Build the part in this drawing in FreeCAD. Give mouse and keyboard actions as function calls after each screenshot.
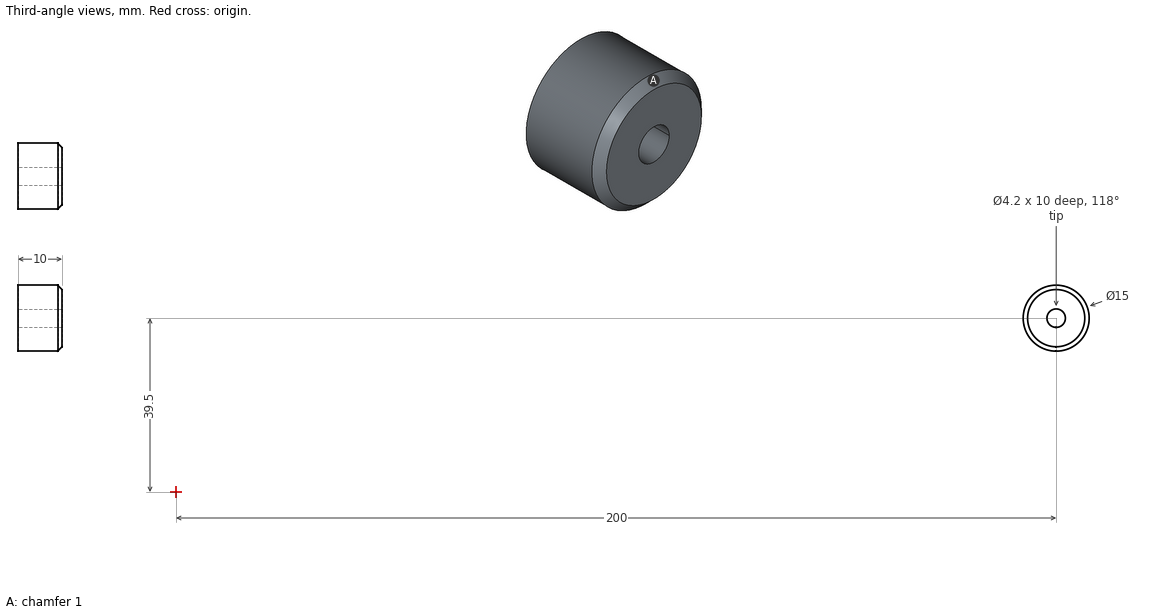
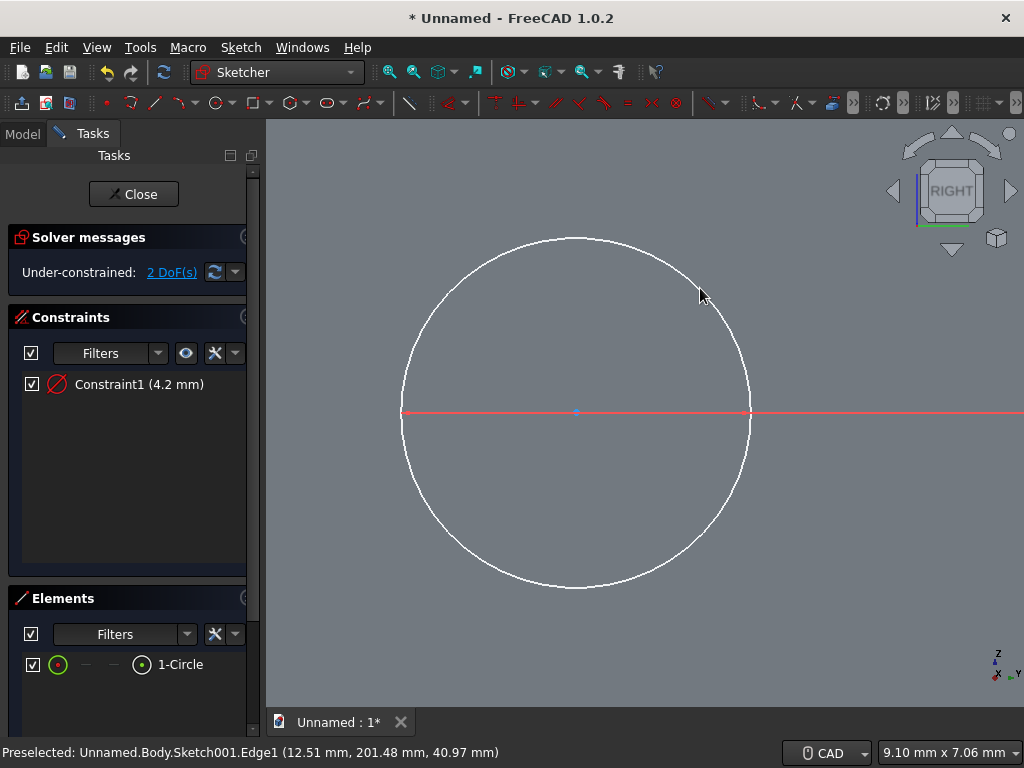
click(448, 104)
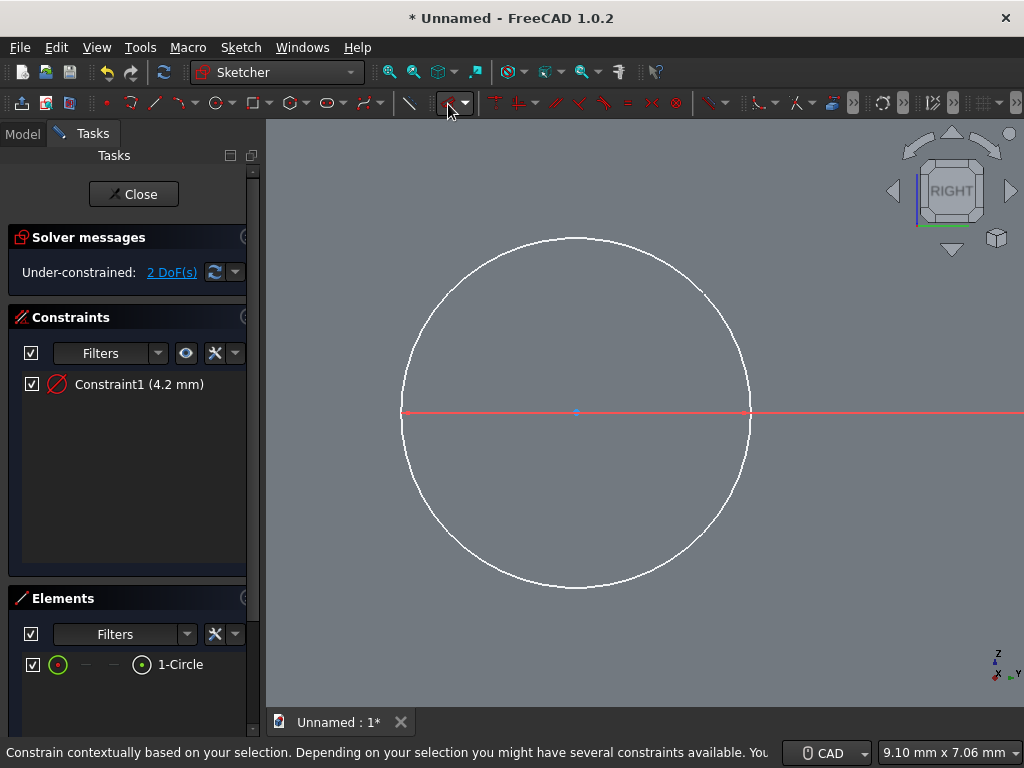
click(576, 413)
click(435, 379)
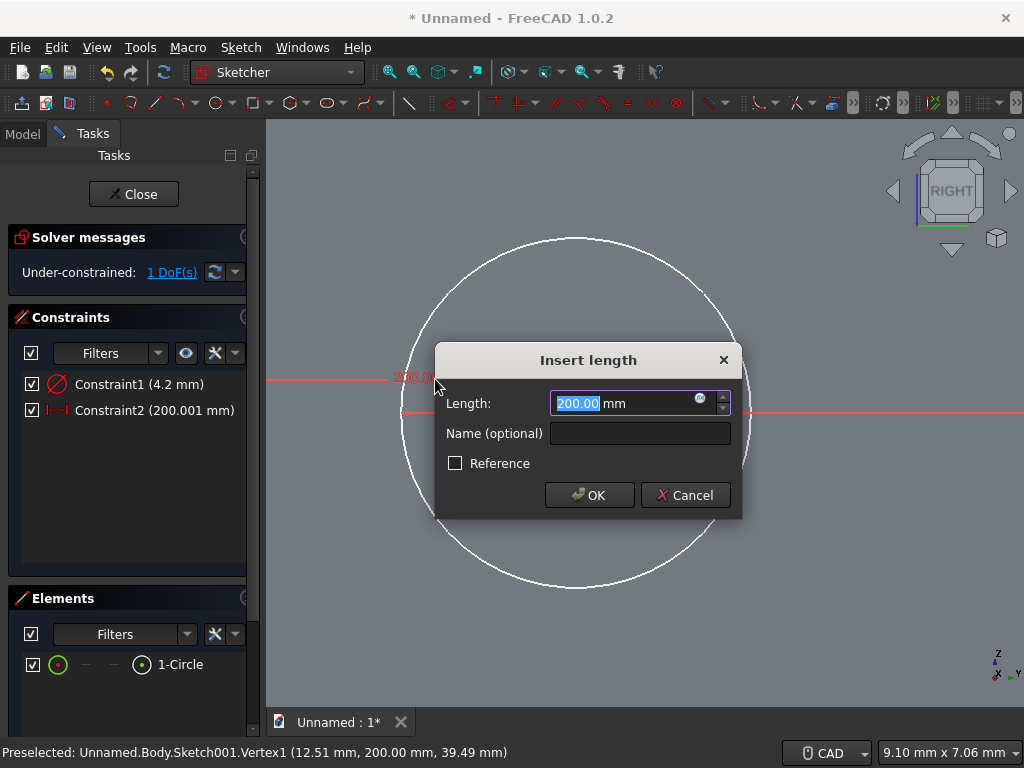
text(200)
key(Return)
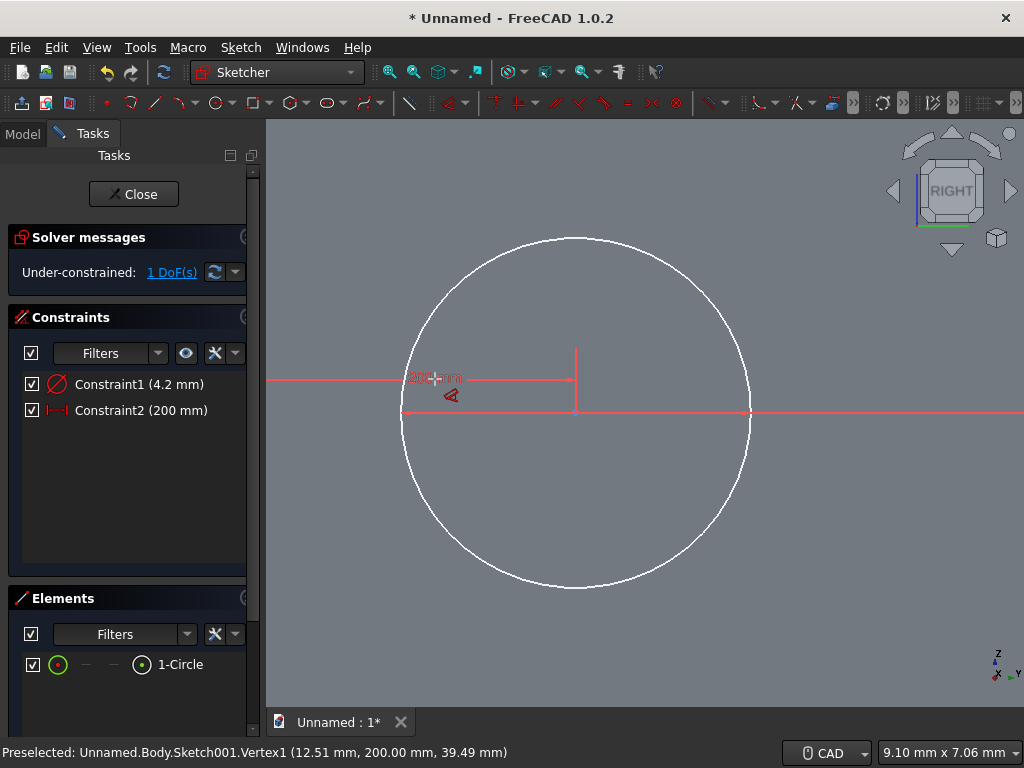
click(576, 413)
click(610, 546)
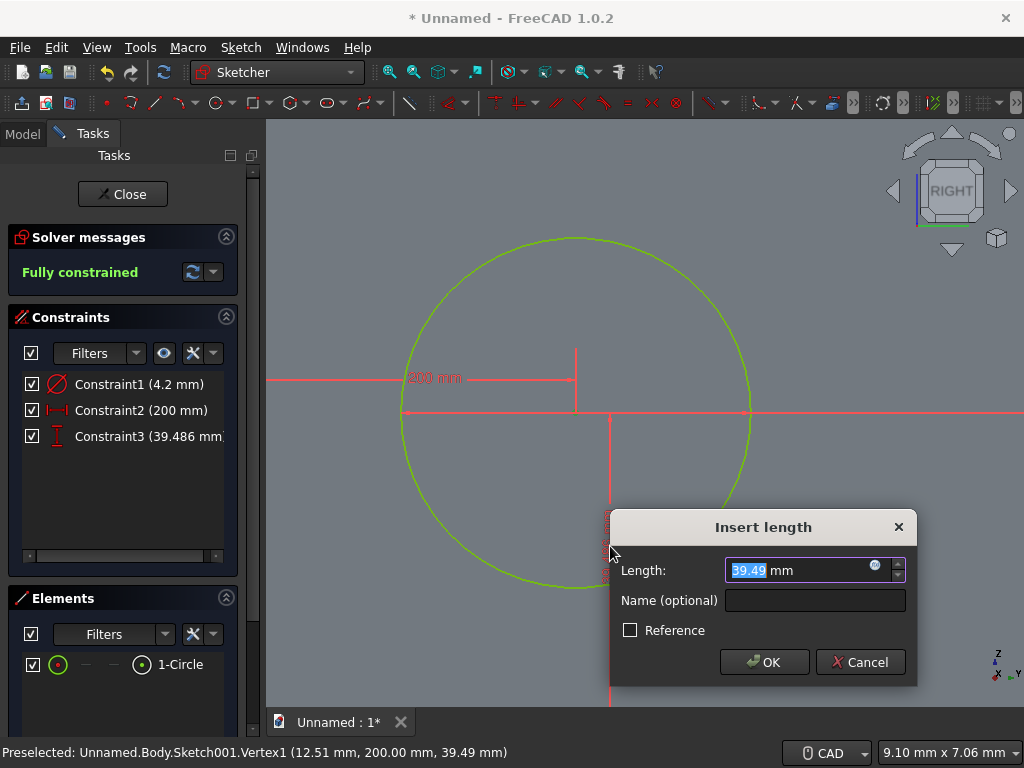
text(39.5)
key(Return)
key(Escape)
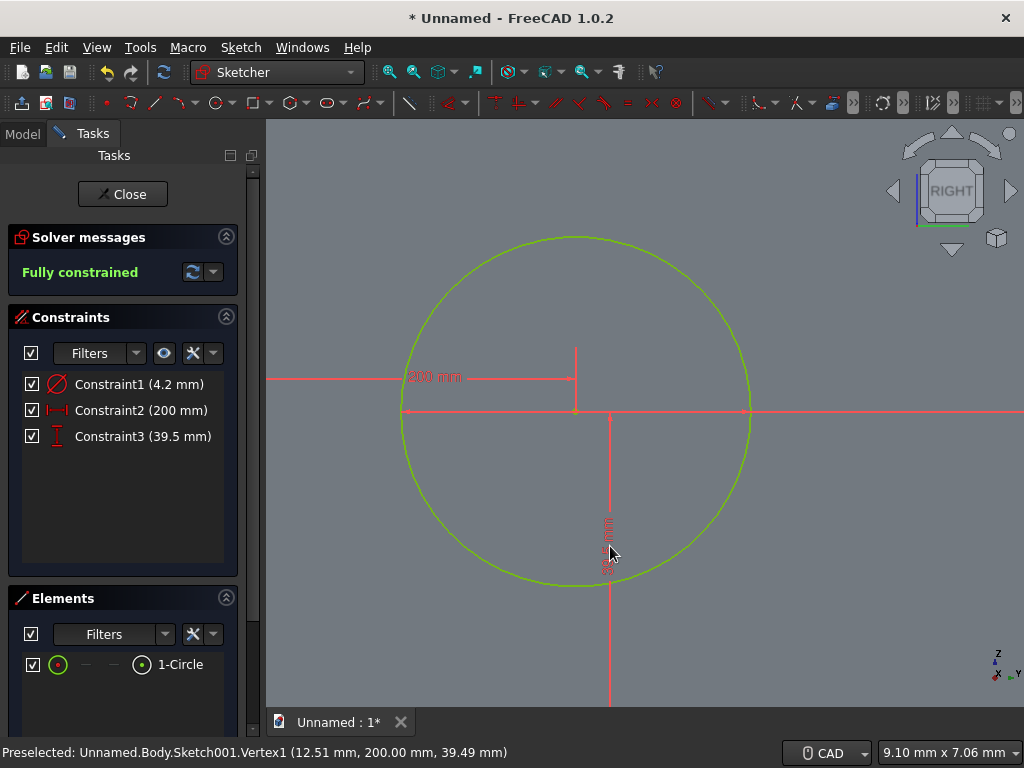
click(123, 194)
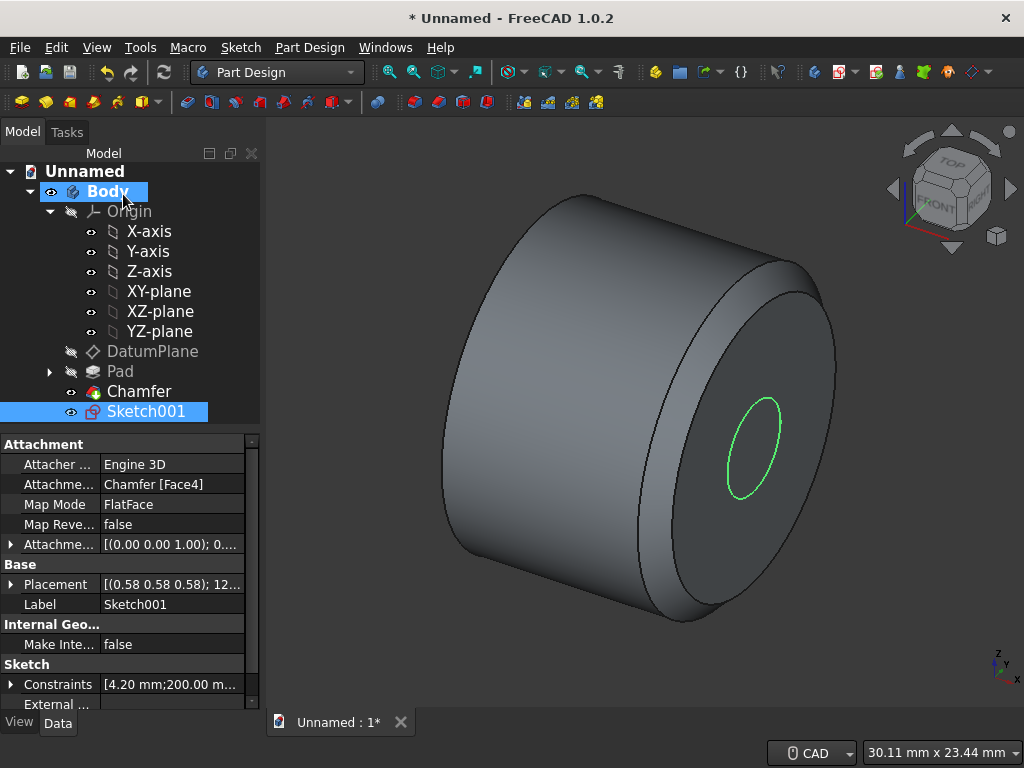
click(212, 102)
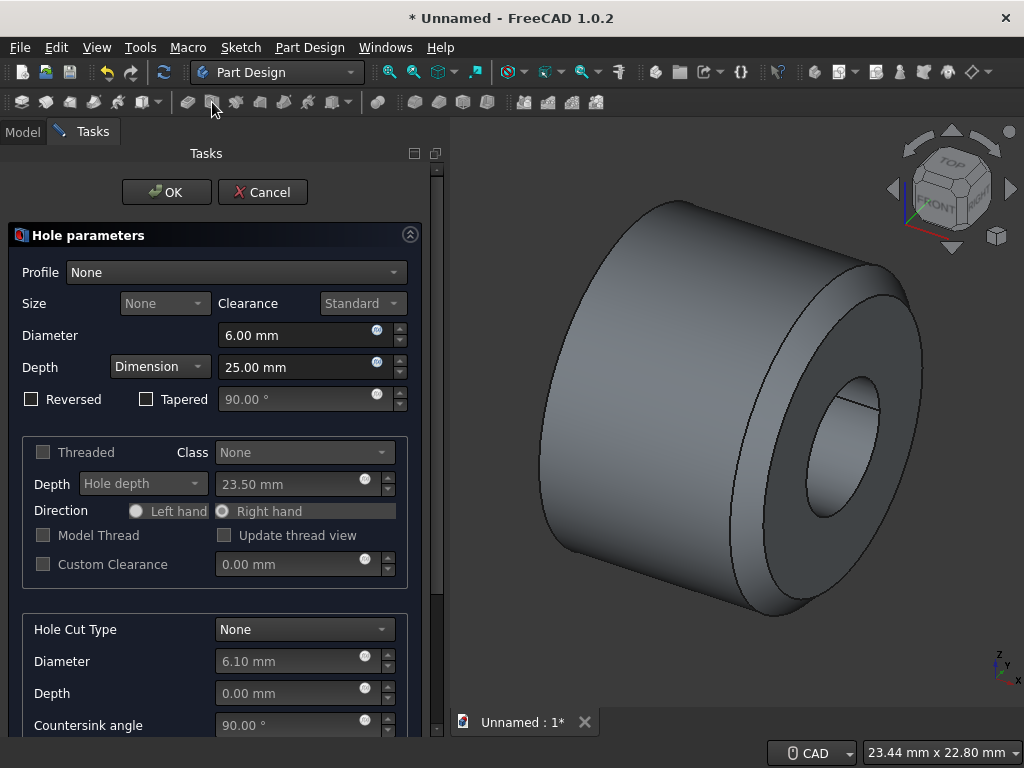
triple_click(305, 335)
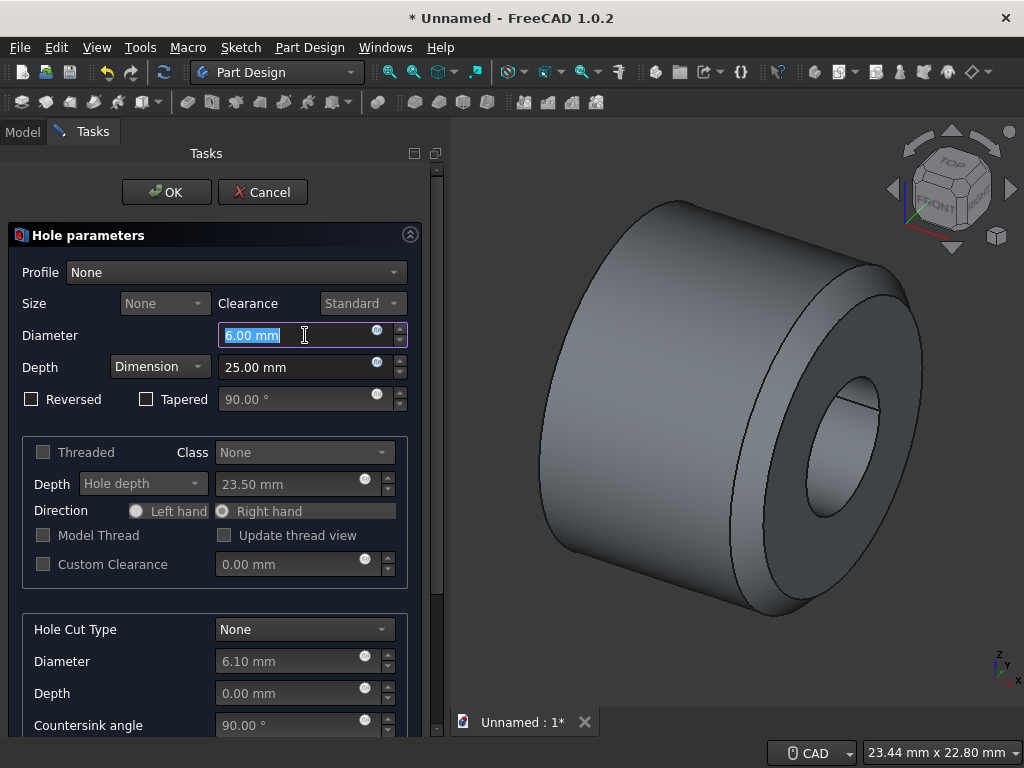
text(4.2)
key(Tab)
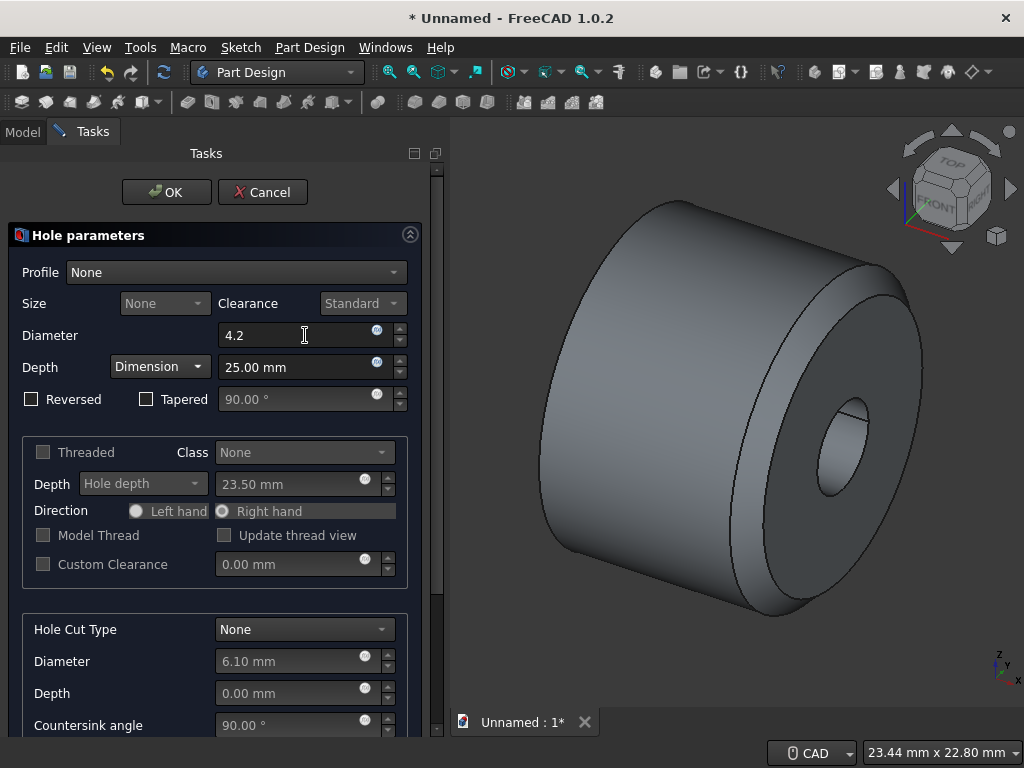
triple_click(305, 367)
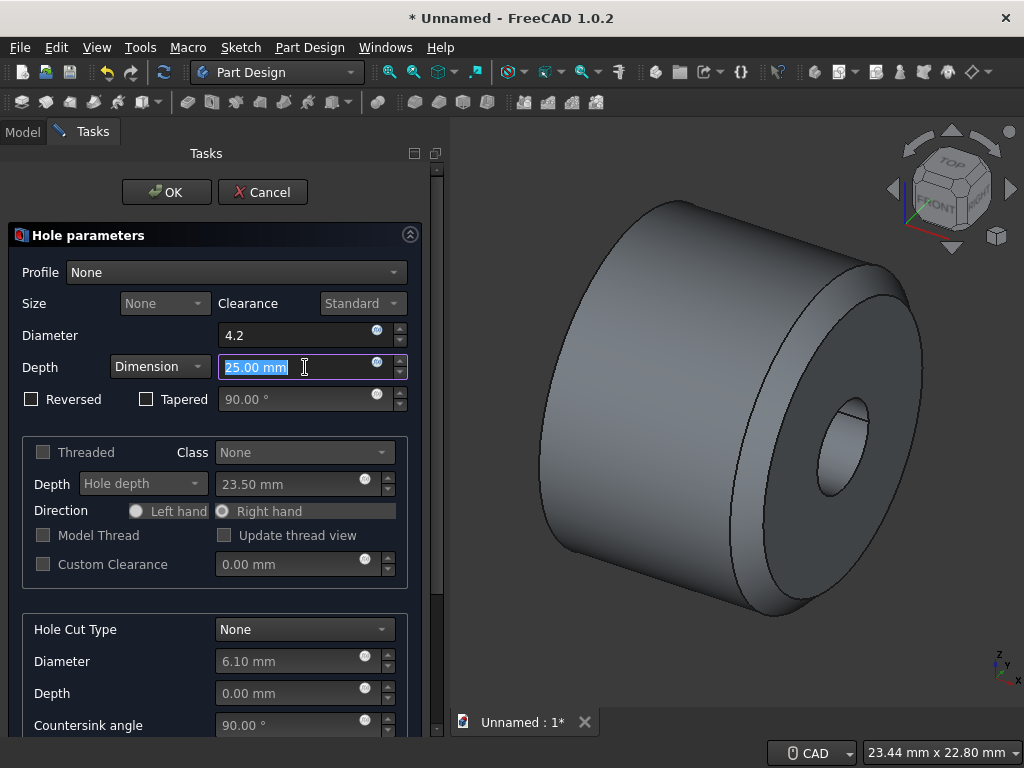
text(10)
key(Tab)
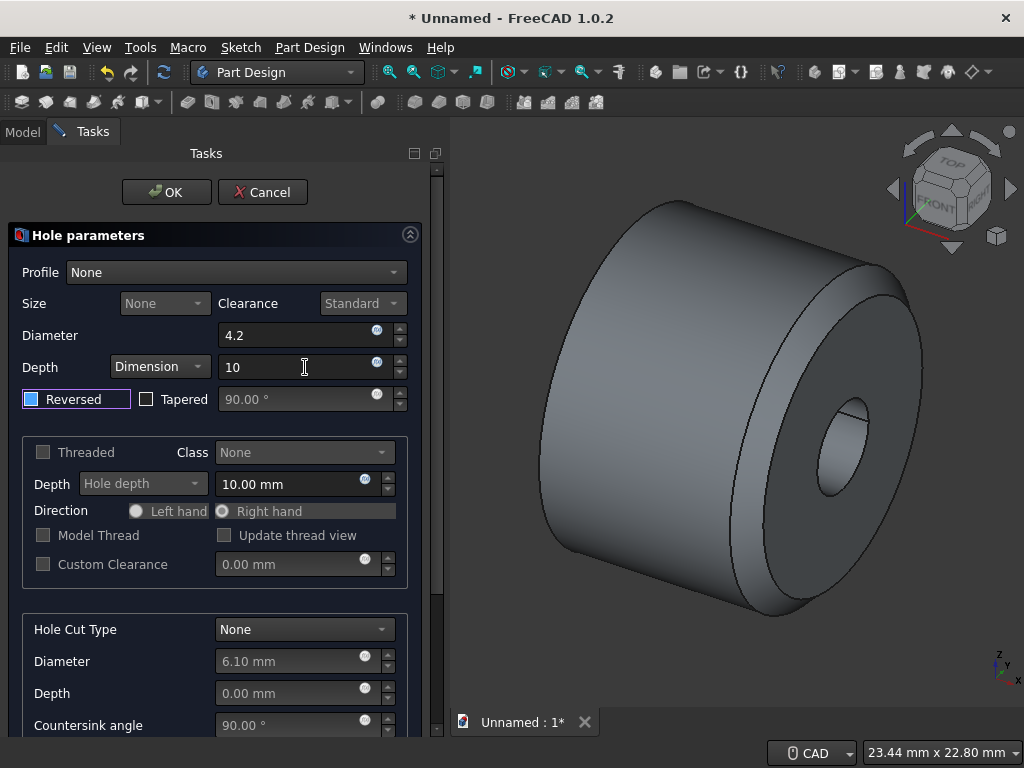
click(167, 192)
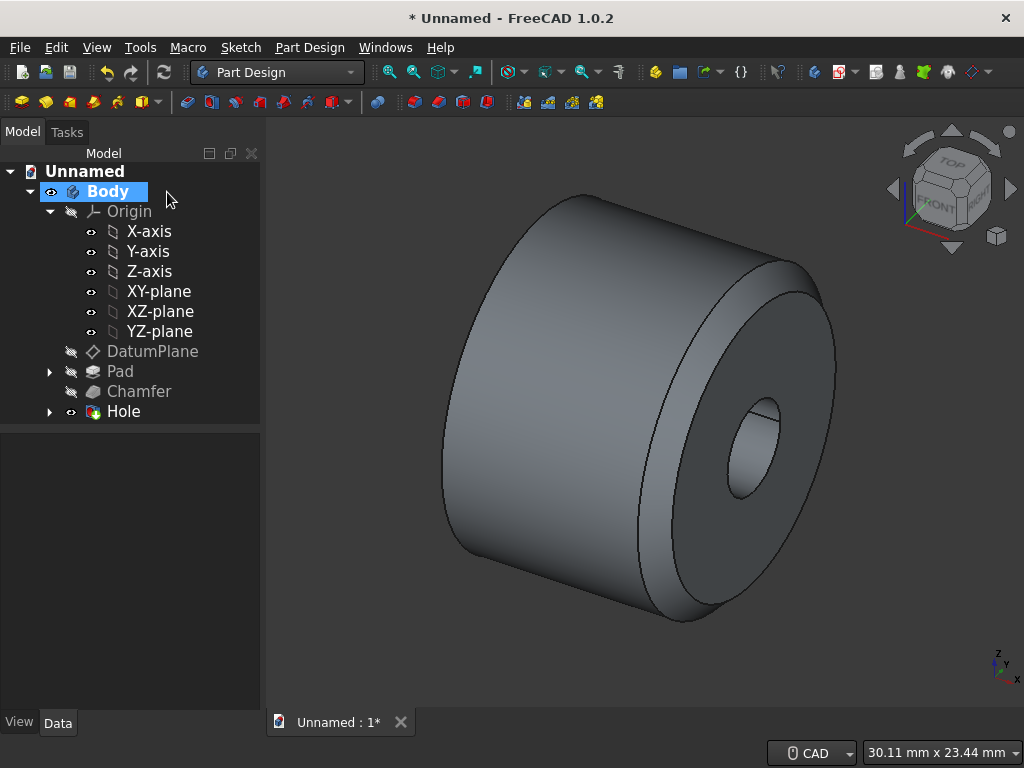
key(0)